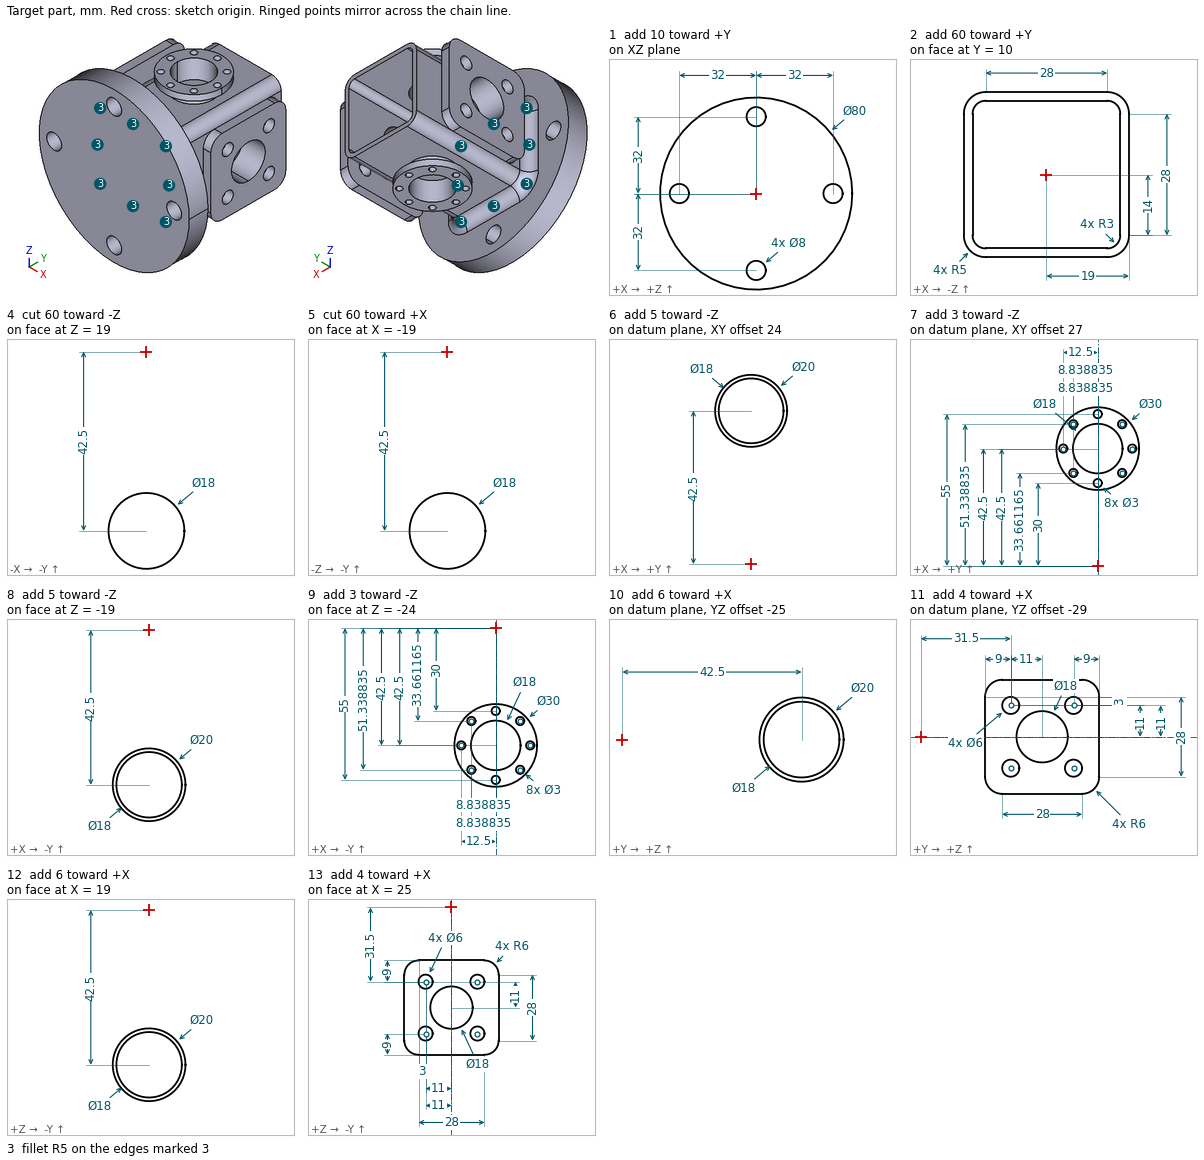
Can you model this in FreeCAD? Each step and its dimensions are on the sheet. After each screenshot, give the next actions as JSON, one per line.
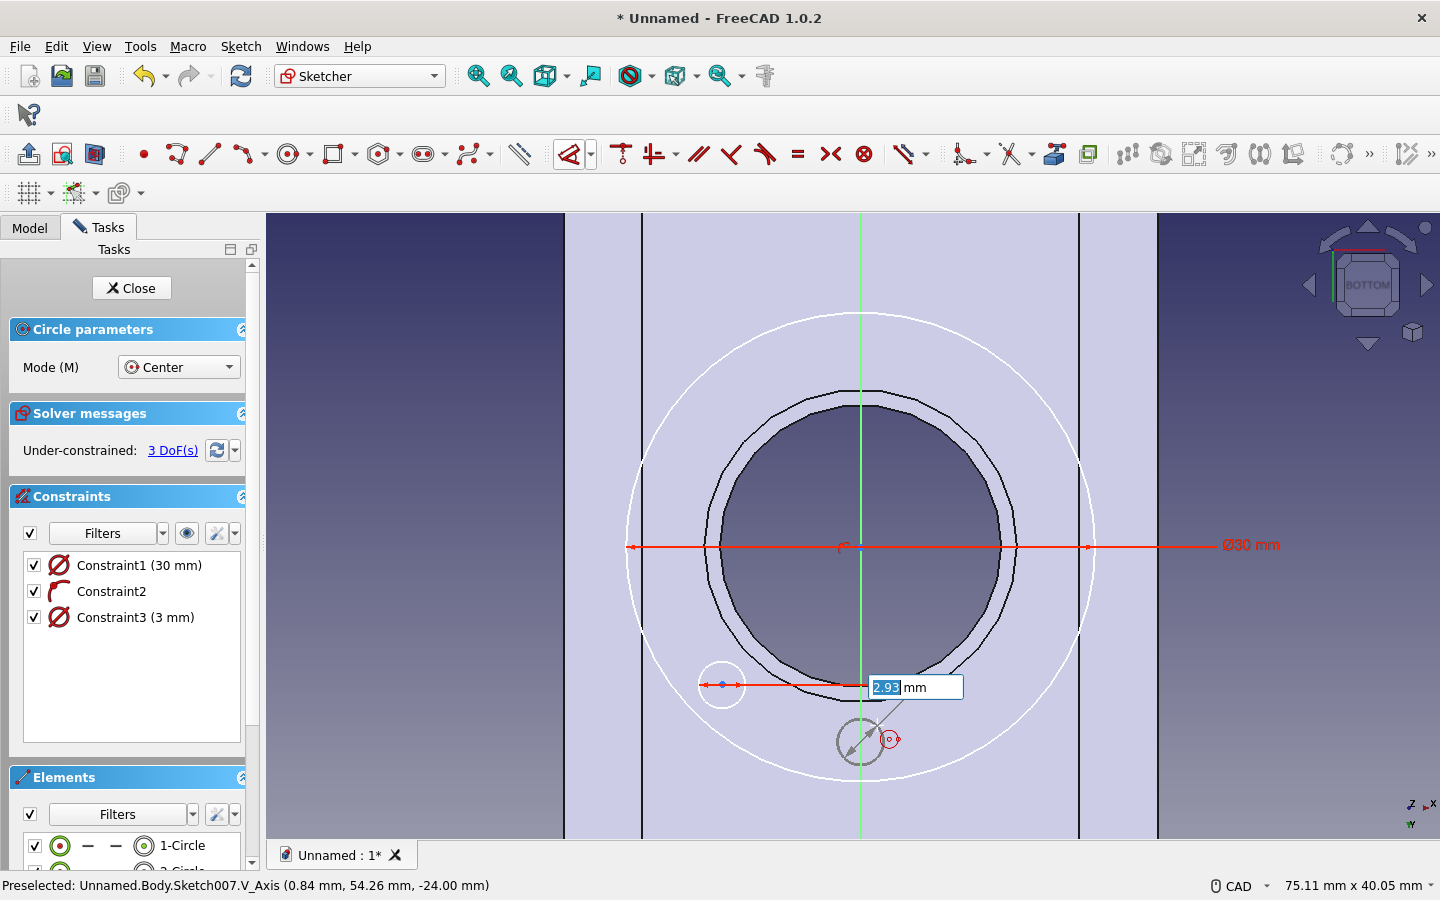
{"action": "type", "text": "3"}
{"action": "key", "text": "Return"}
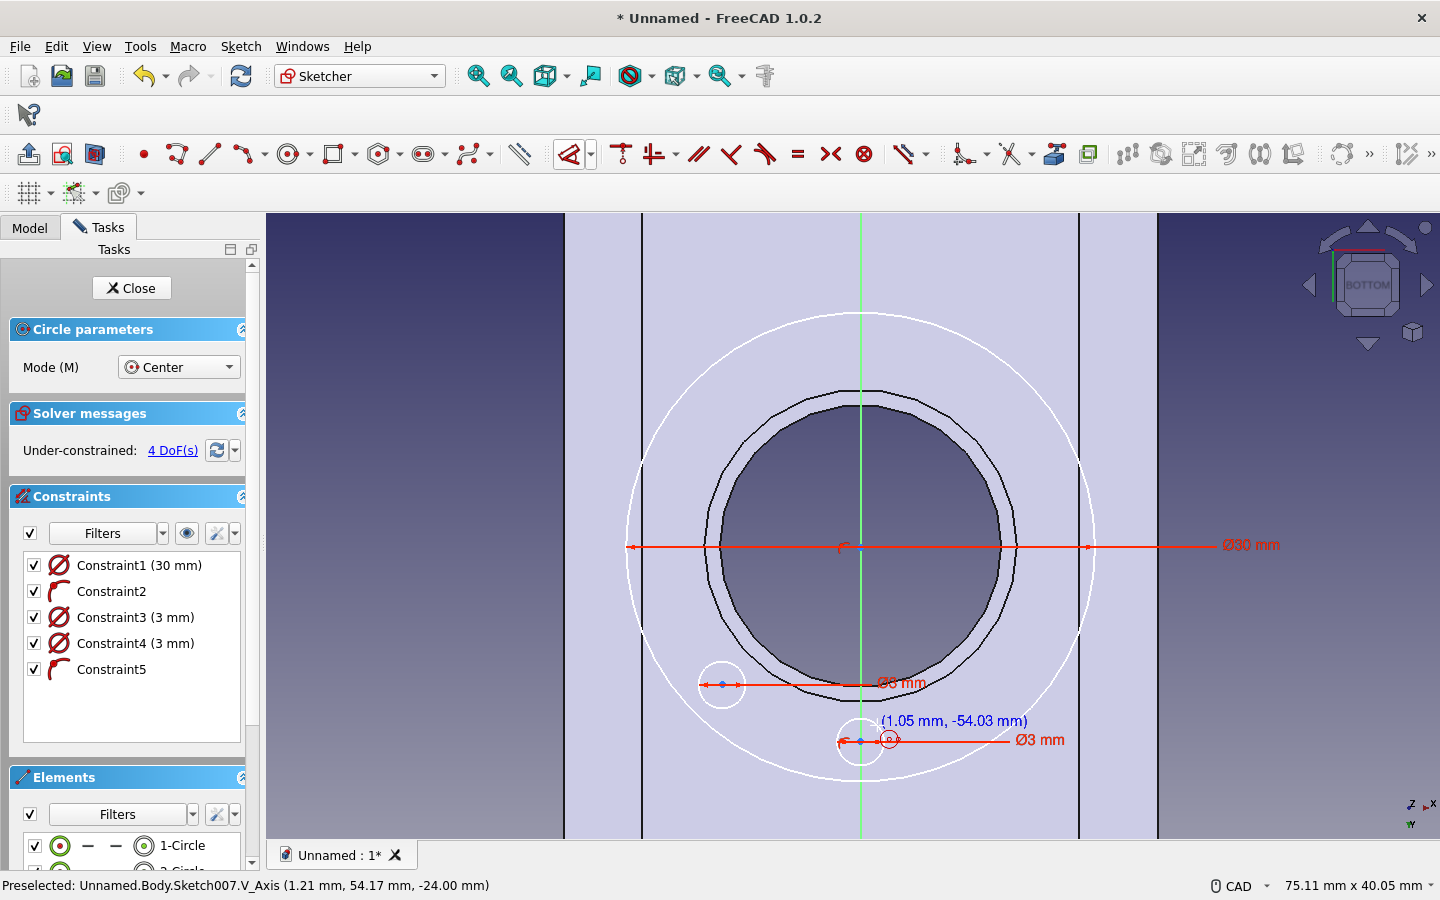
{"action": "left_click", "coordinate": [999, 684]}
{"action": "mouse_move", "coordinate": [1015, 667]}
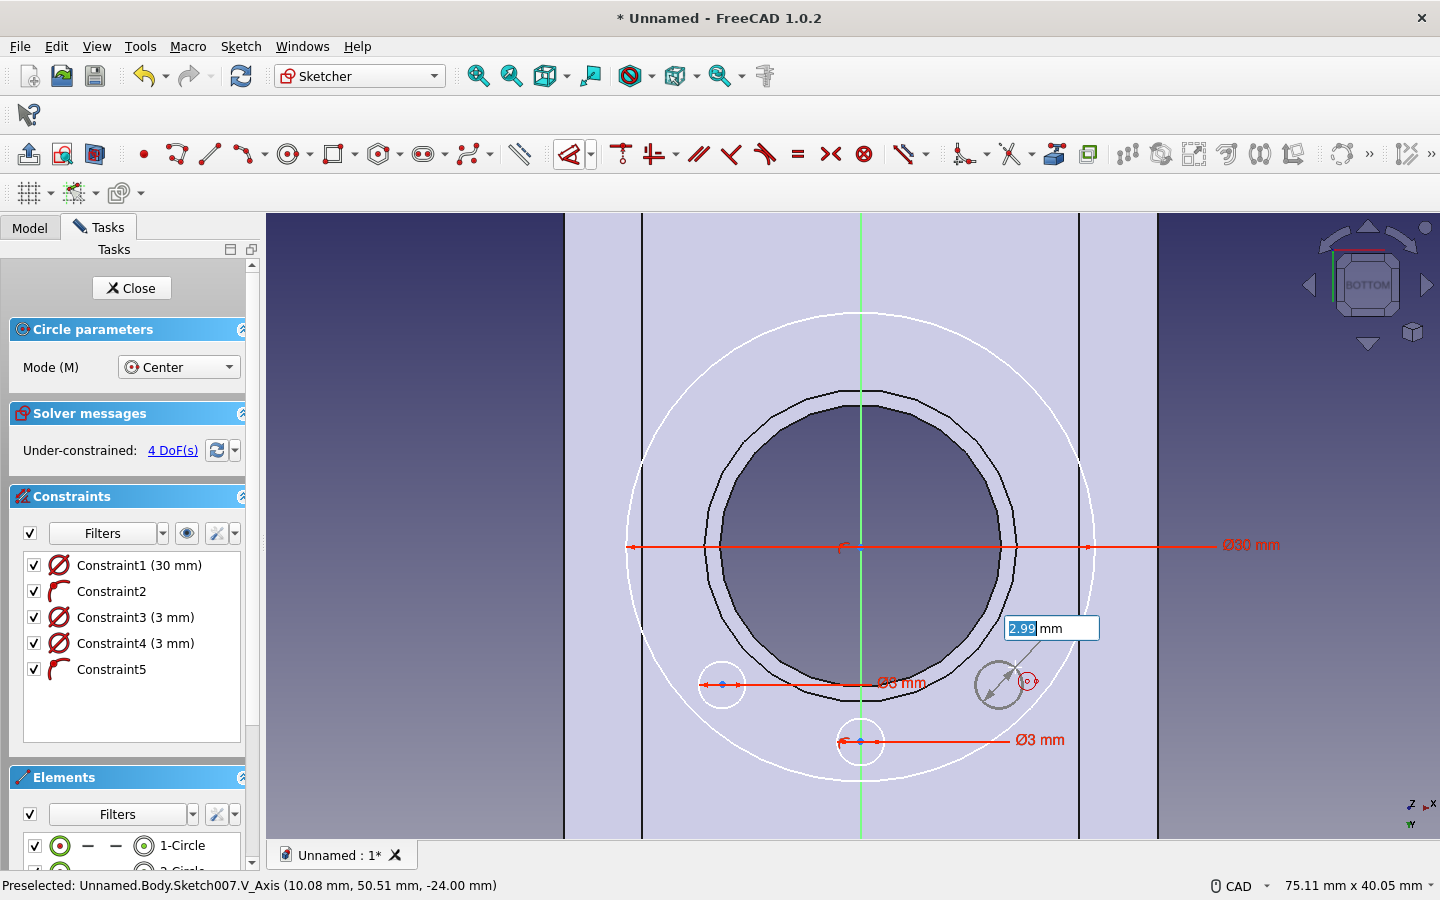
{"action": "type", "text": "3"}
{"action": "key", "text": "Return"}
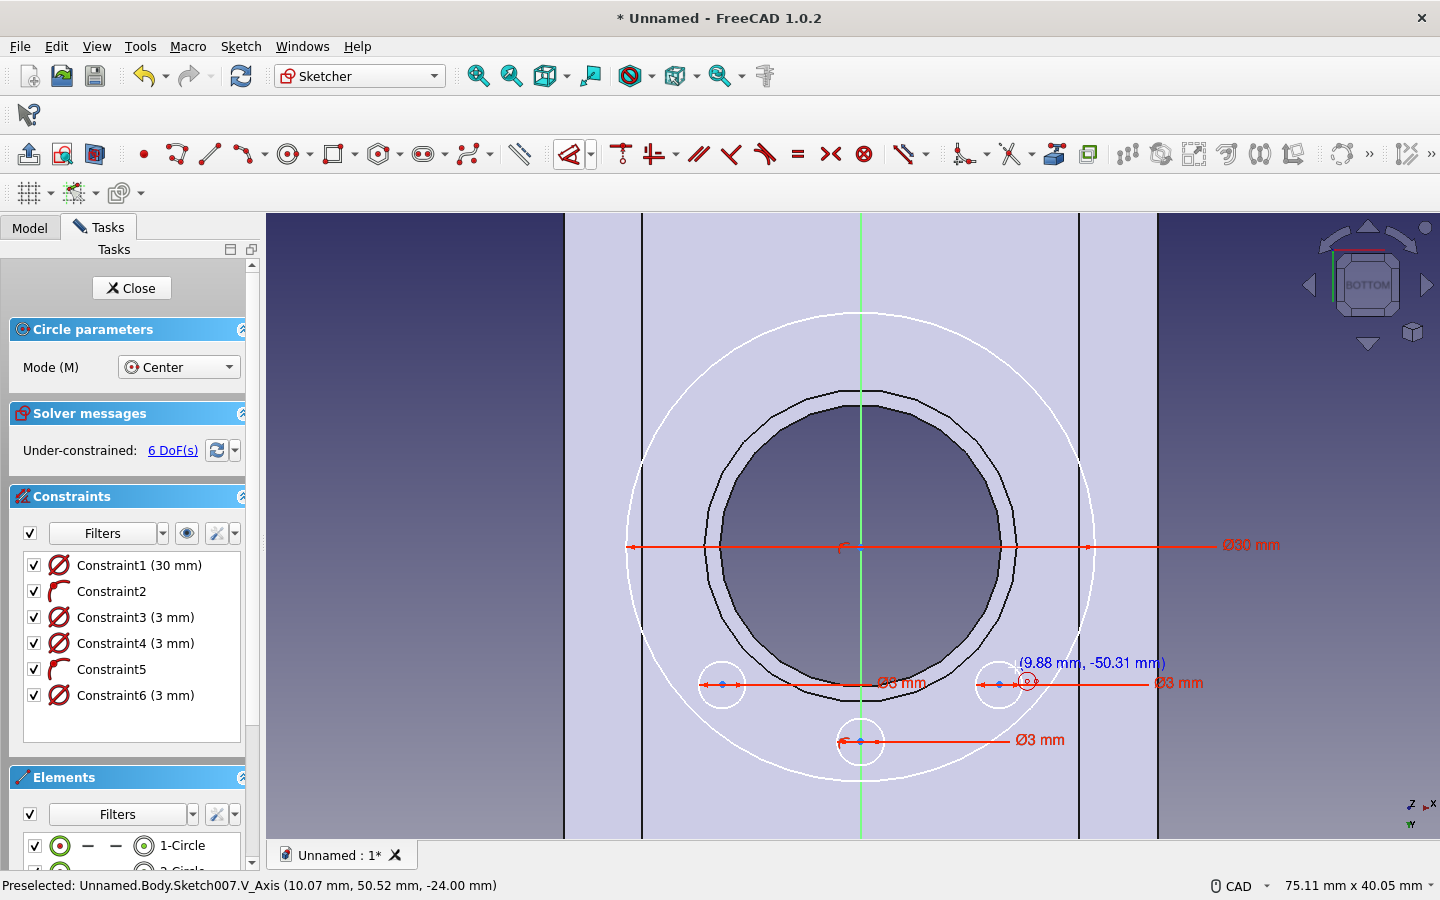
{"action": "left_click", "coordinate": [665, 546]}
{"action": "mouse_move", "coordinate": [682, 529]}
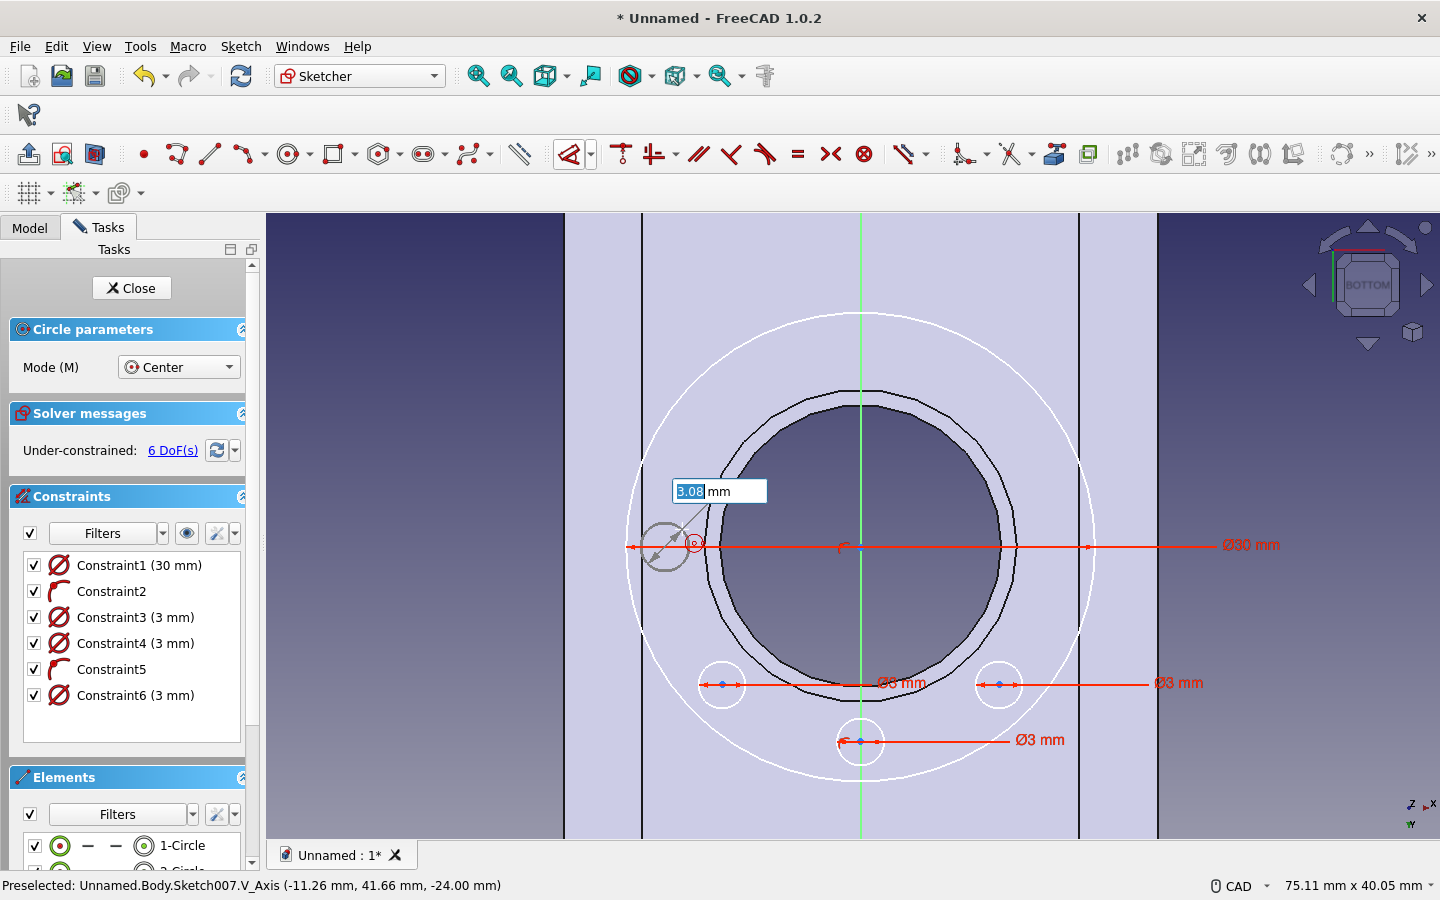
{"action": "type", "text": "3"}
{"action": "key", "text": "Return"}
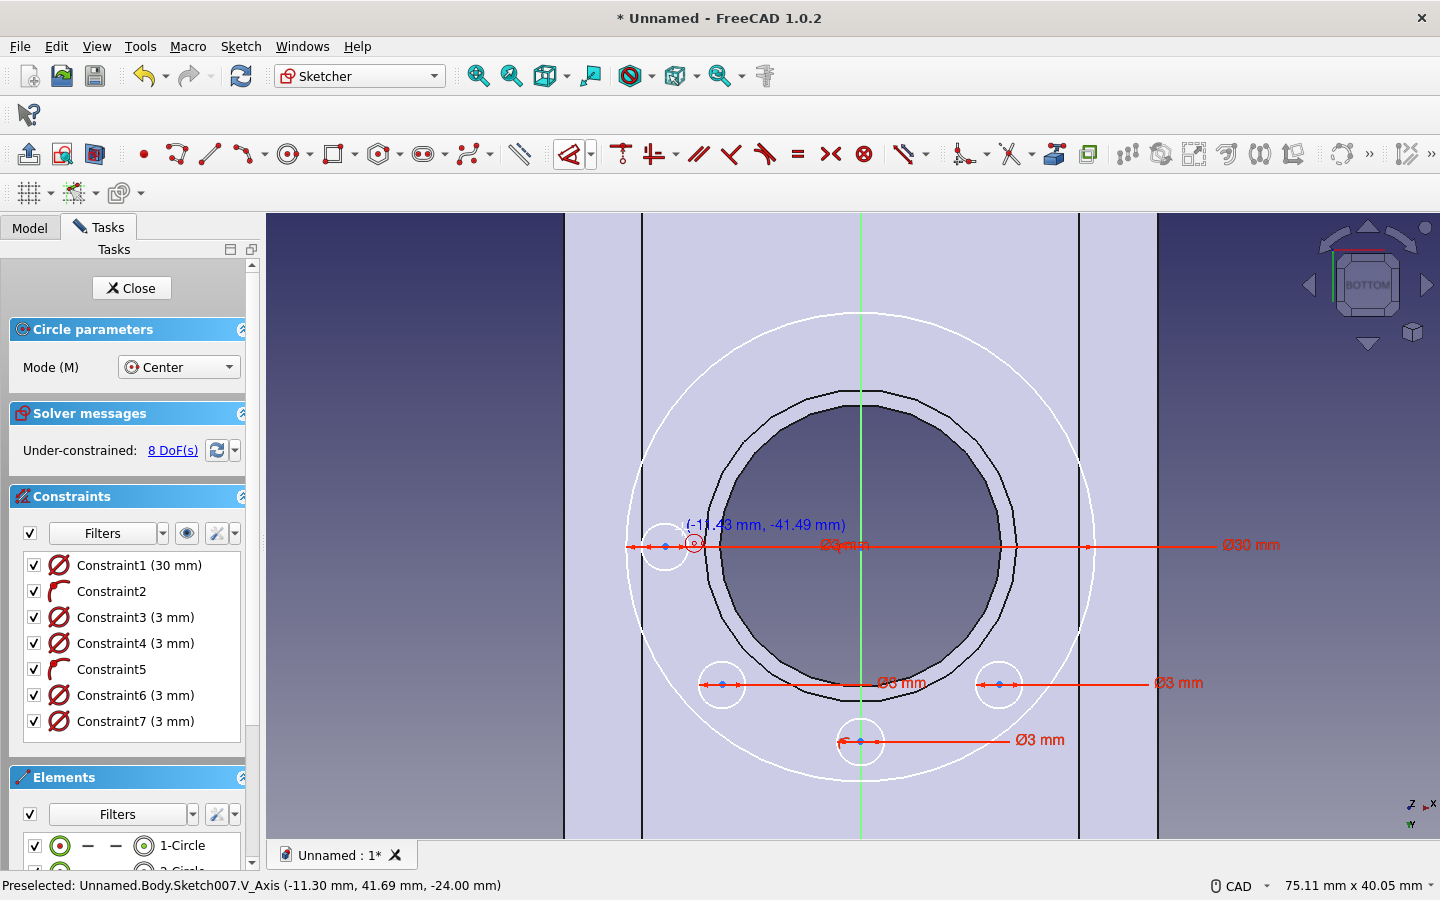
{"action": "left_click", "coordinate": [722, 408]}
{"action": "mouse_move", "coordinate": [739, 391]}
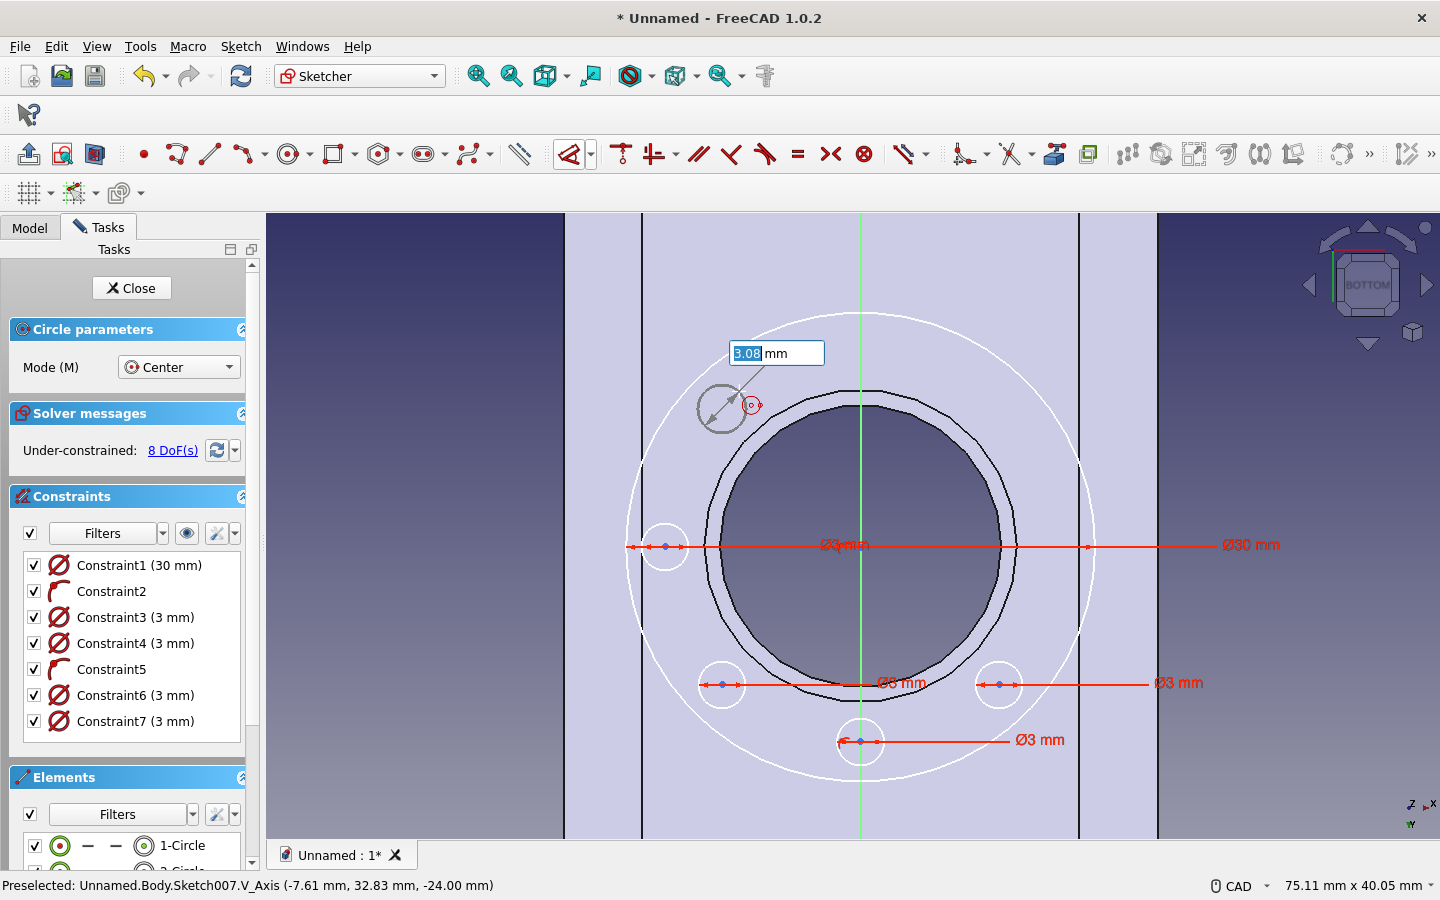
{"action": "type", "text": "3"}
{"action": "key", "text": "Return"}